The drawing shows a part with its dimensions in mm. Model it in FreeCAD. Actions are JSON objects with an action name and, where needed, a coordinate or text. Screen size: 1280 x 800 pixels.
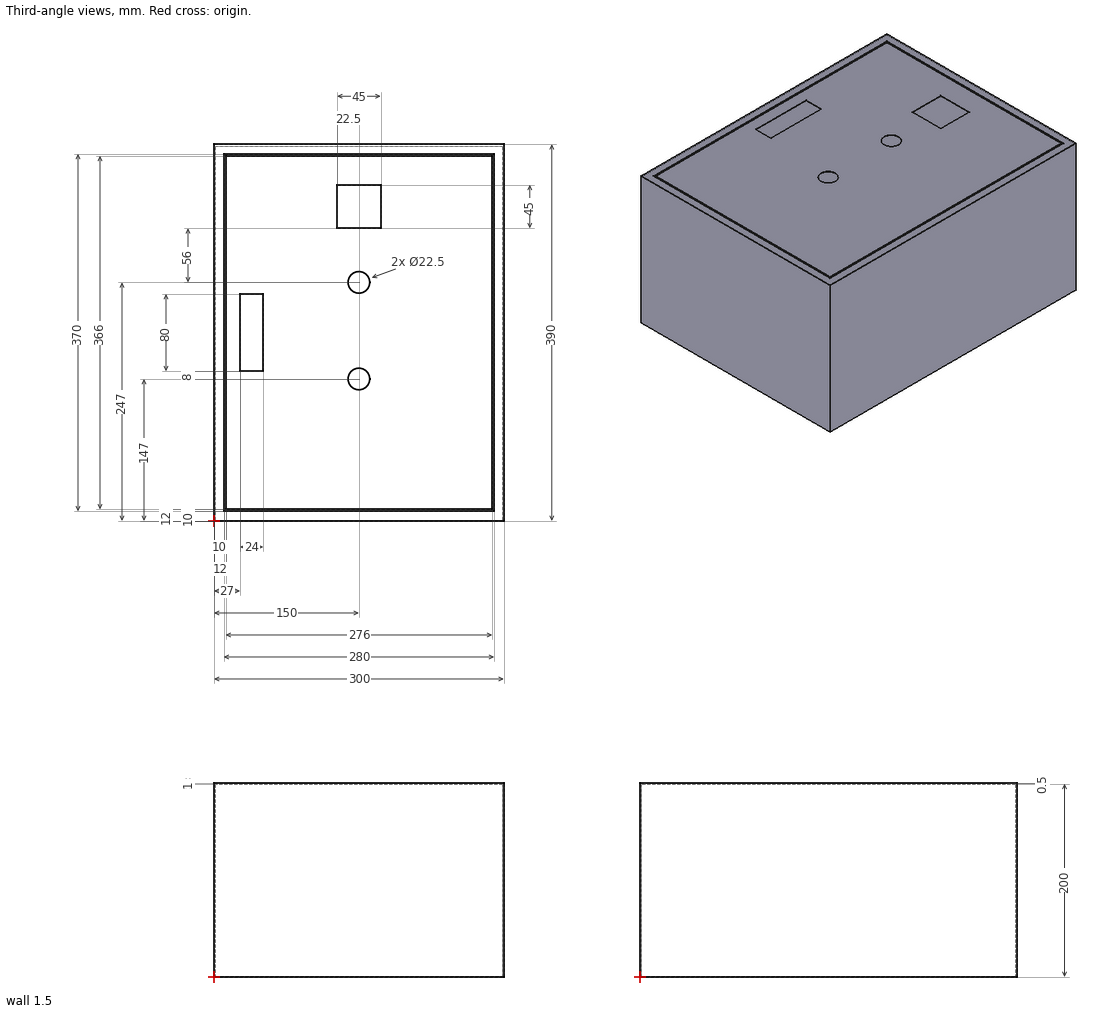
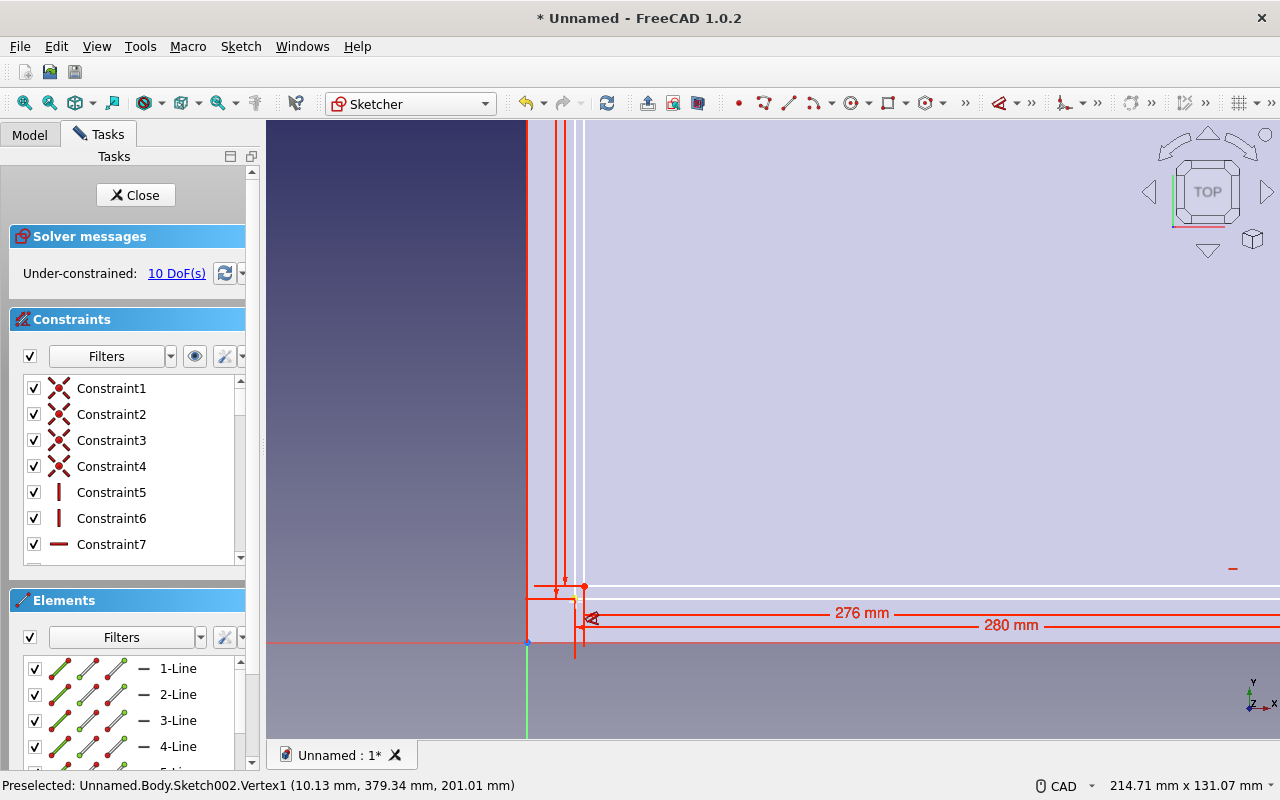
{"action": "left_click", "coordinate": [575, 599]}
{"action": "left_click", "coordinate": [493, 621]}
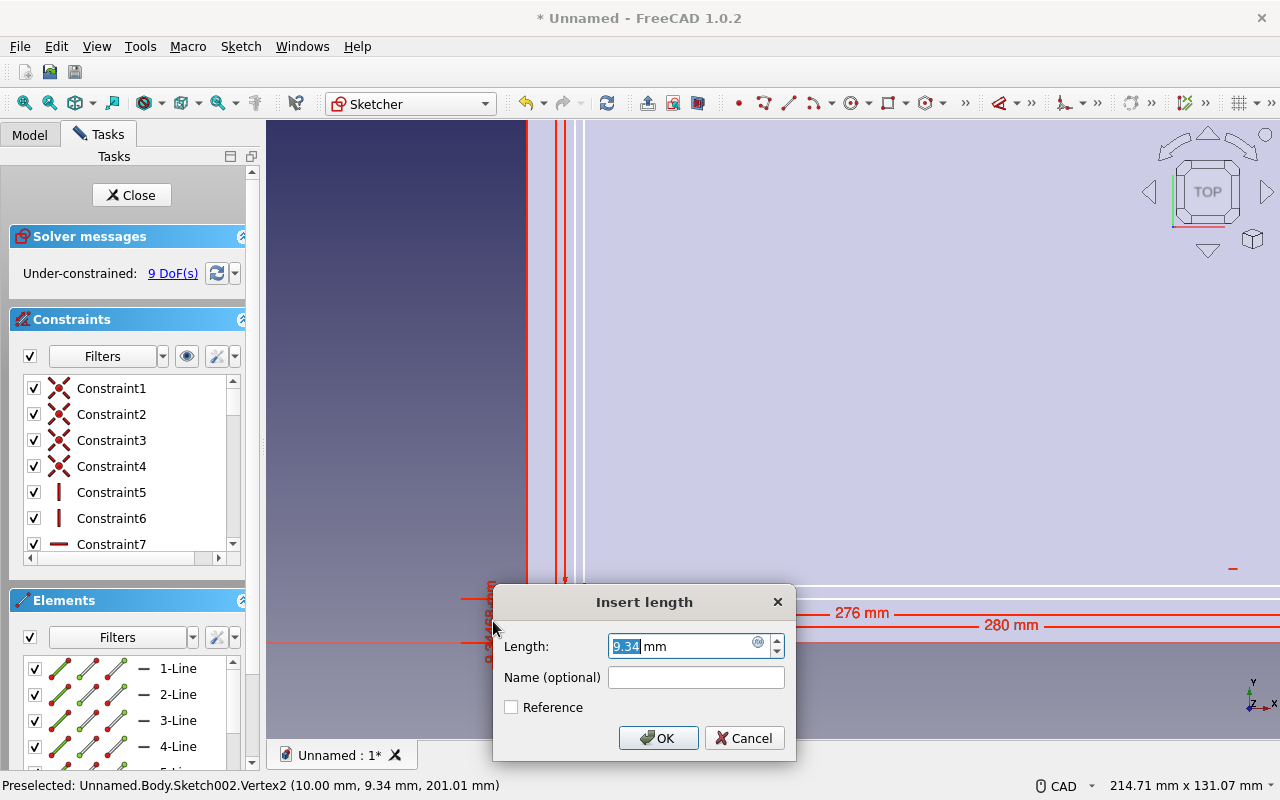
{"action": "type", "text": "10"}
{"action": "key", "text": "Return"}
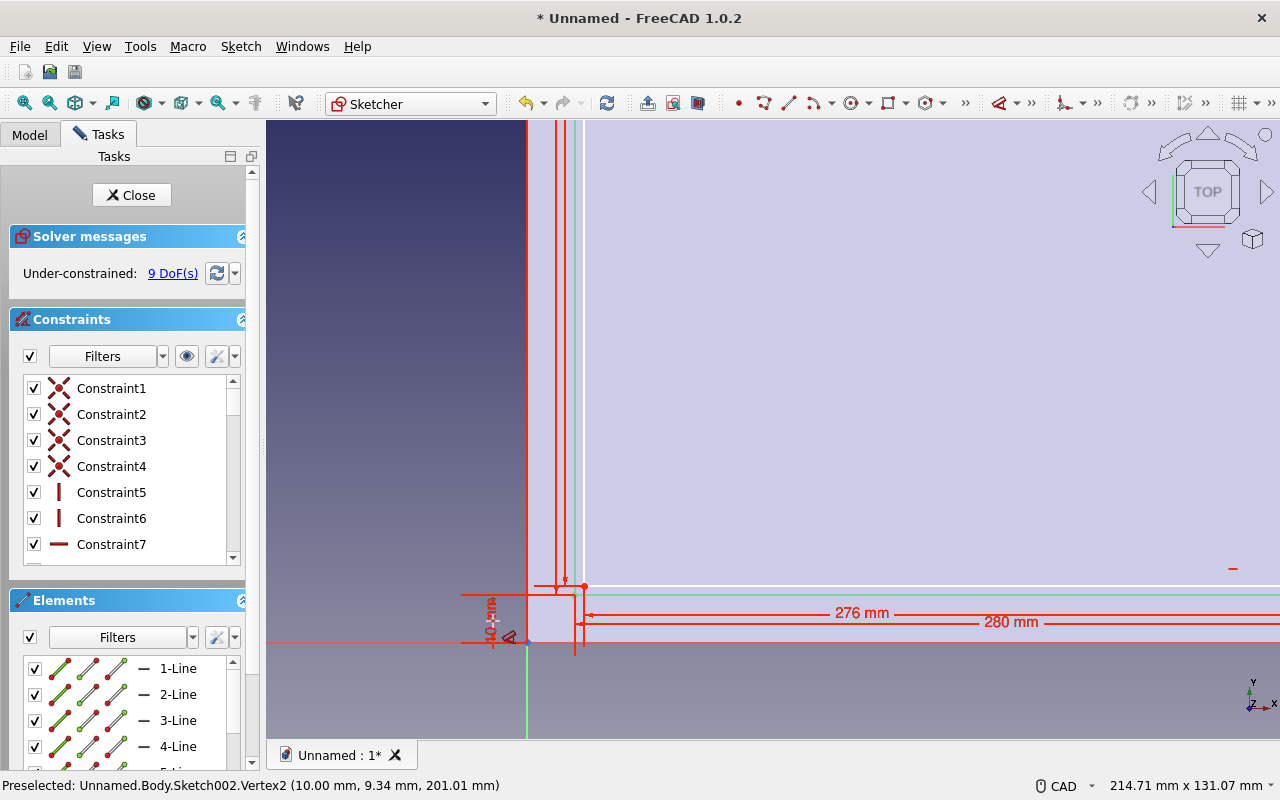
{"action": "scroll", "coordinate": [576, 603], "scroll_direction": "down", "scroll_amount": 8}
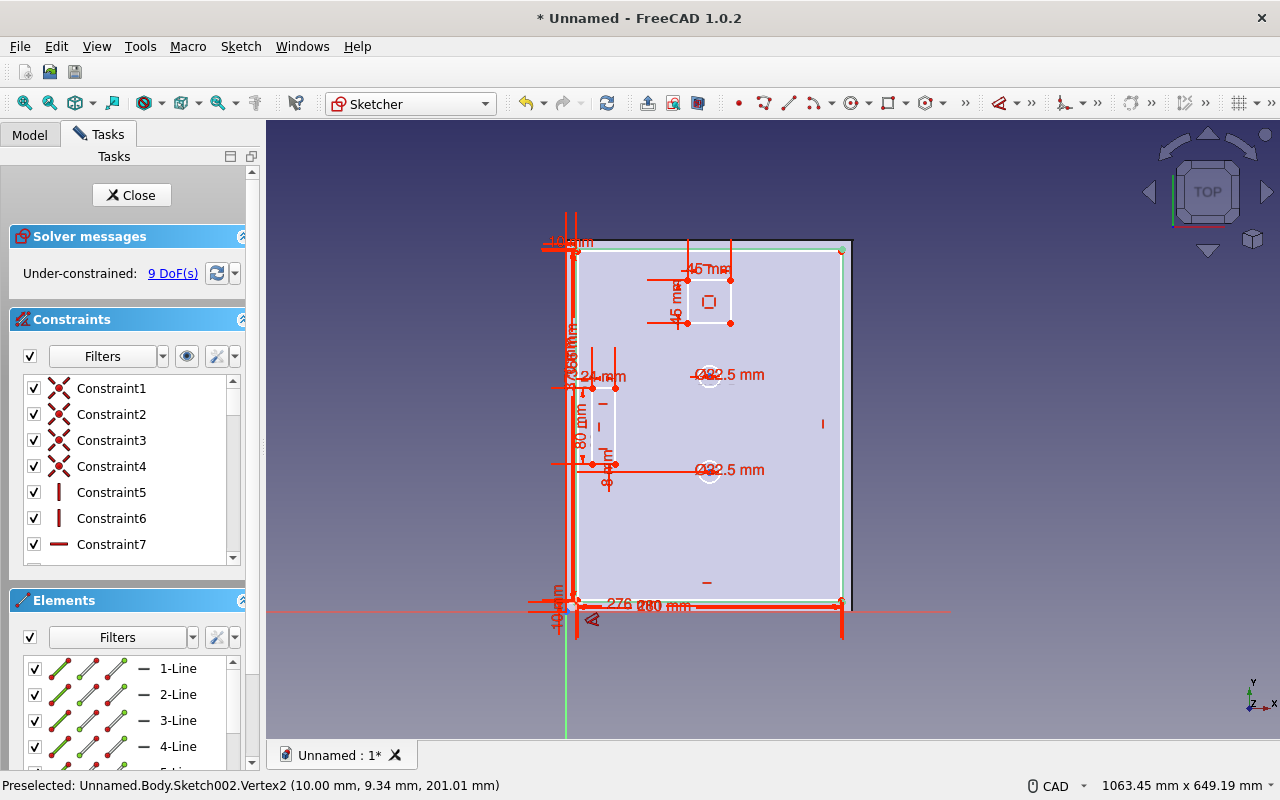
{"action": "scroll", "coordinate": [592, 388], "scroll_direction": "up", "scroll_amount": 3}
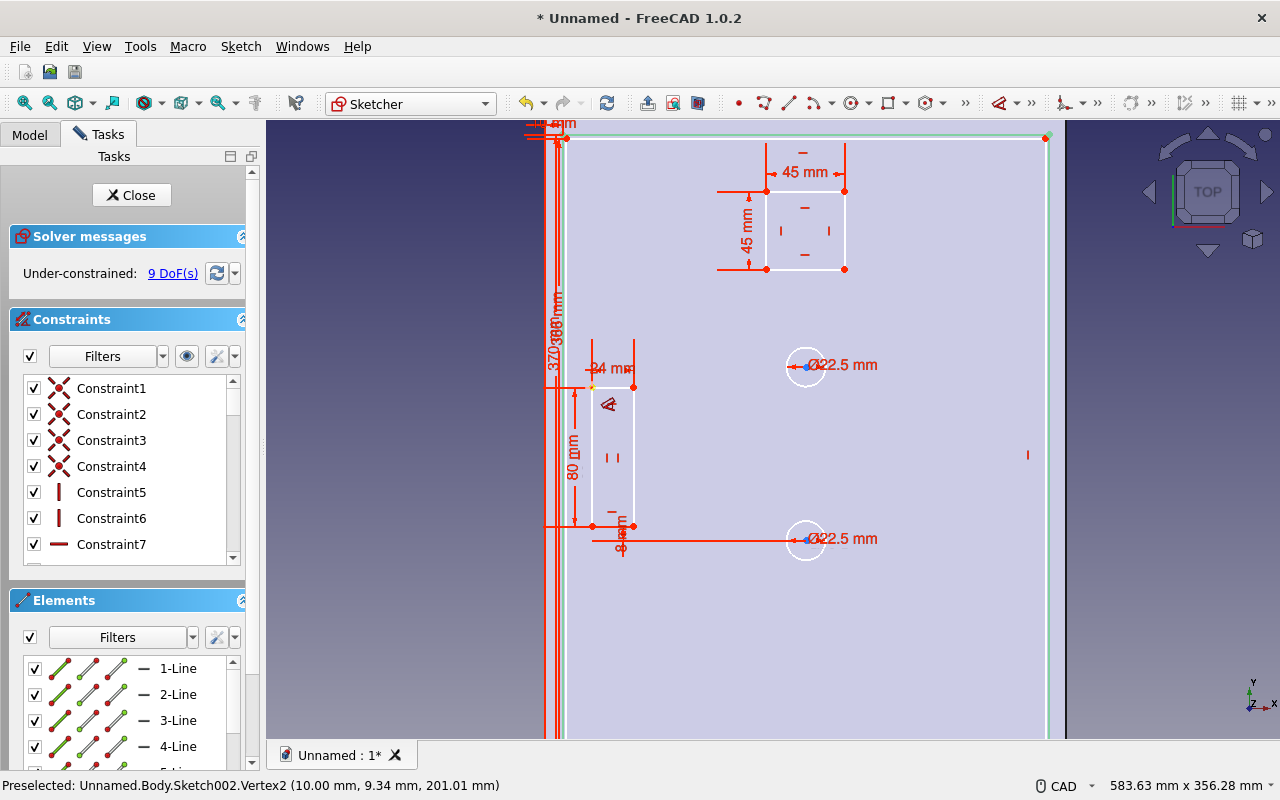
{"action": "left_click", "coordinate": [592, 388]}
{"action": "left_click", "coordinate": [579, 282]}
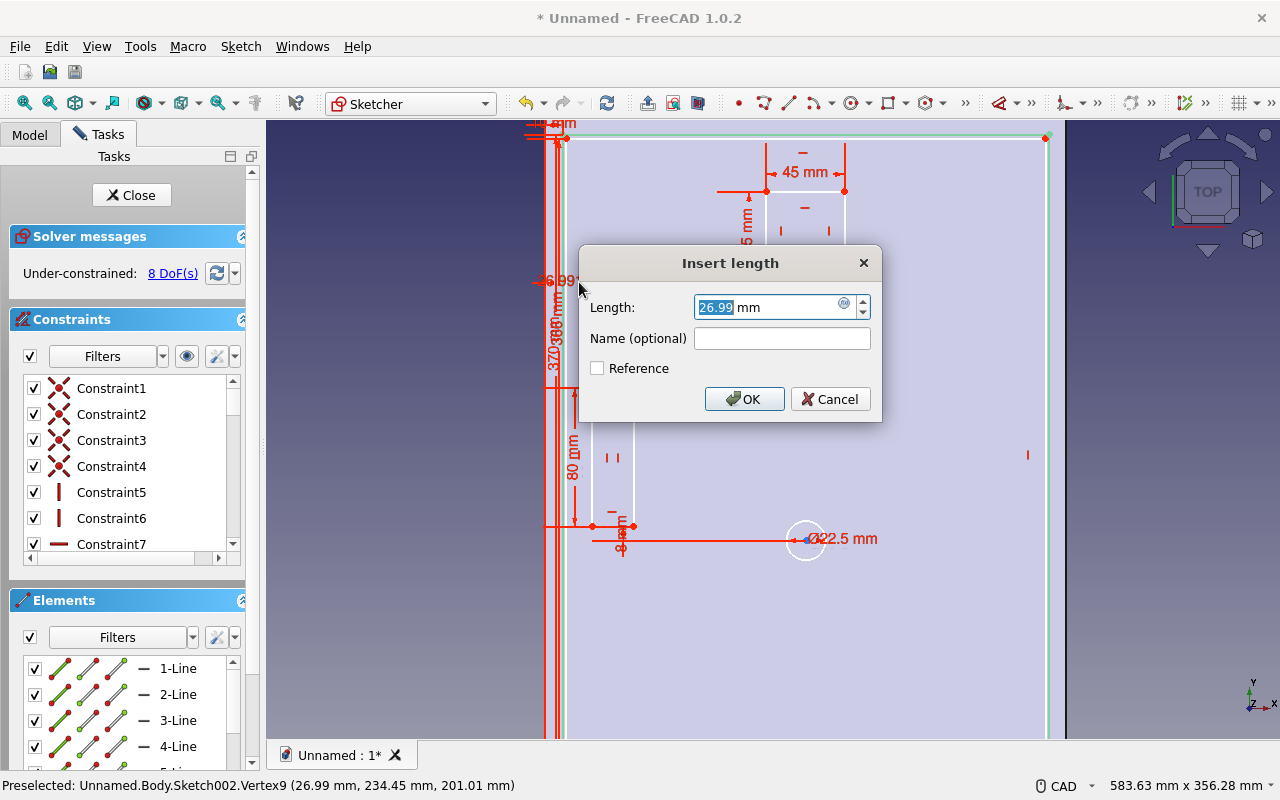
{"action": "type", "text": "27"}
{"action": "key", "text": "Return"}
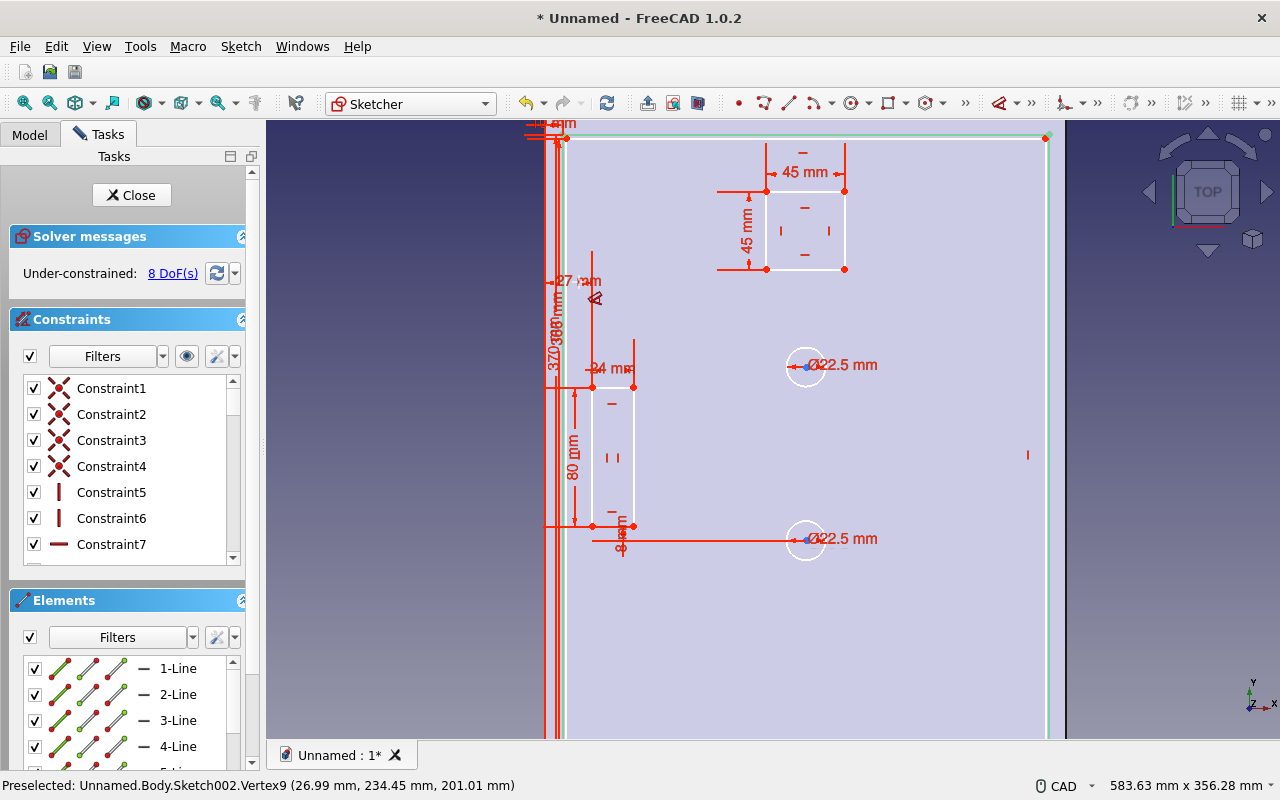
{"action": "scroll", "coordinate": [592, 386], "scroll_direction": "down", "scroll_amount": 3}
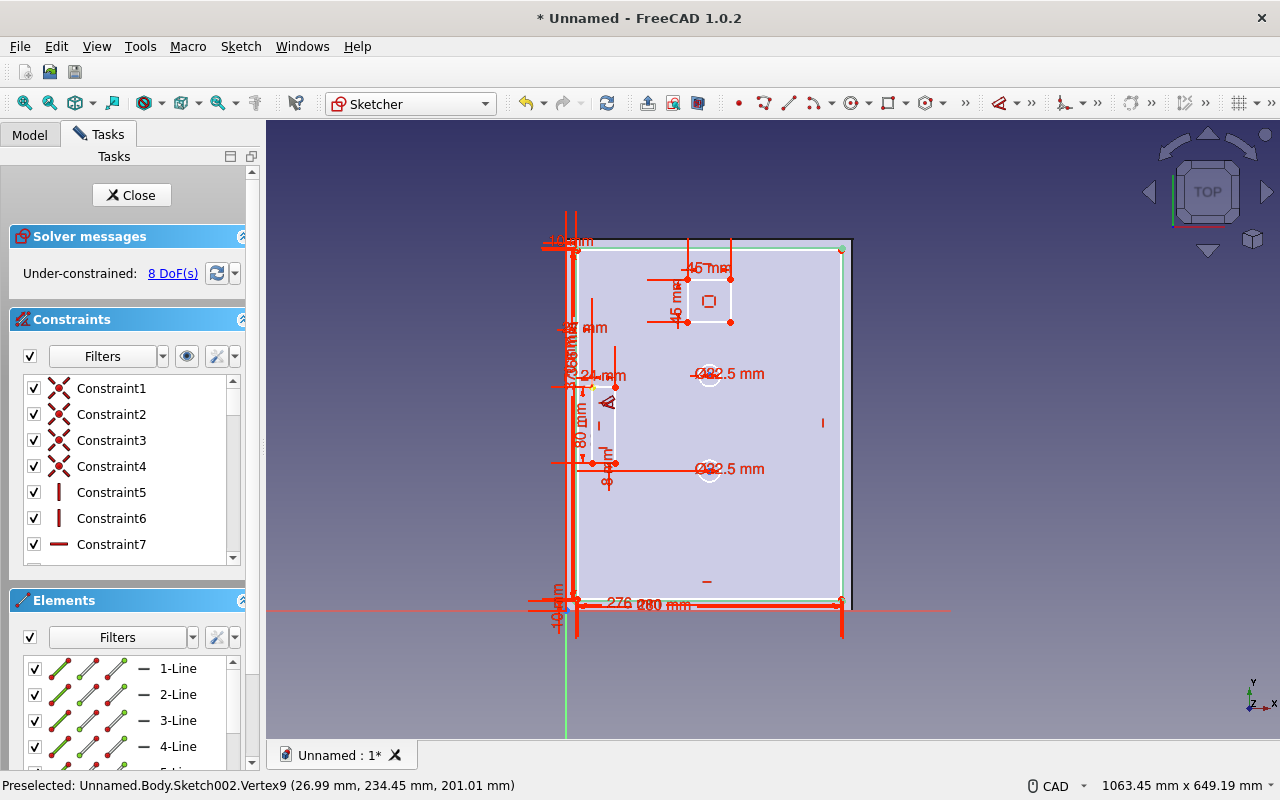
{"action": "scroll", "coordinate": [578, 250], "scroll_direction": "up", "scroll_amount": 8}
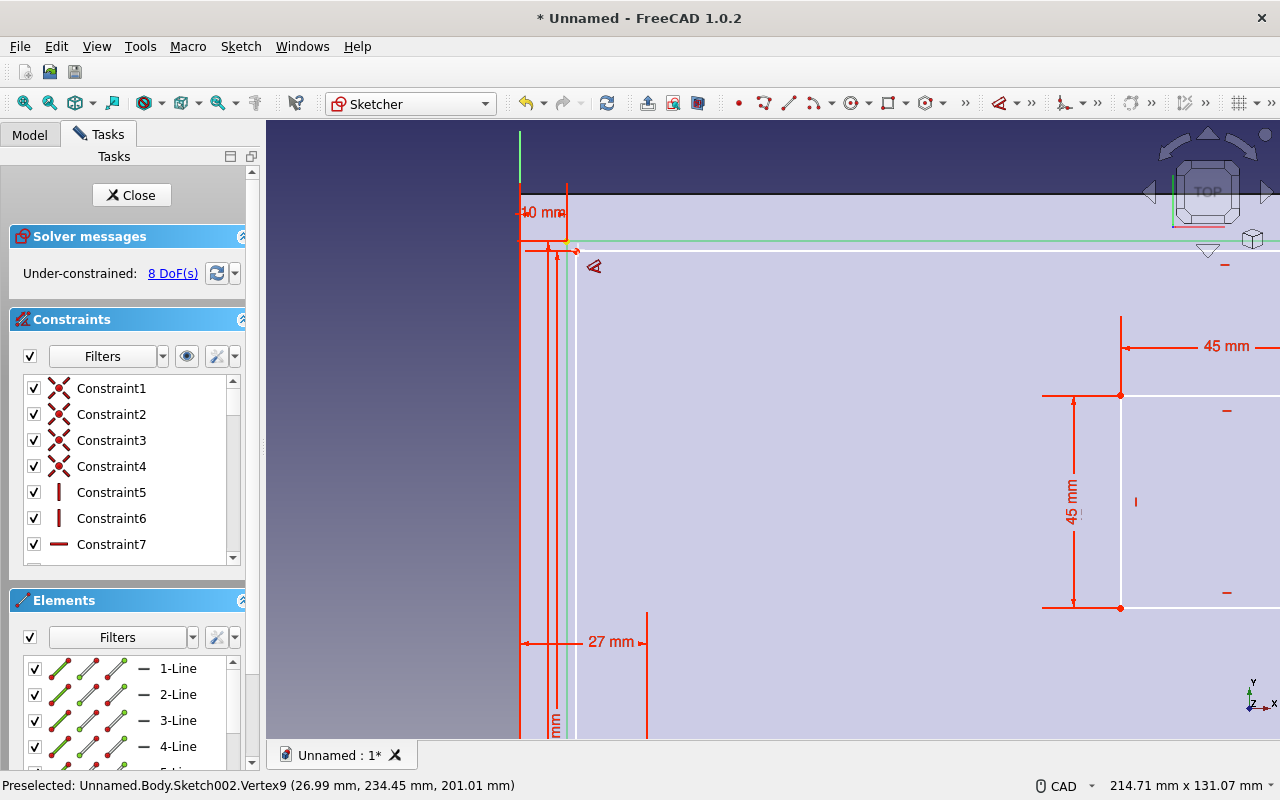
{"action": "left_click", "coordinate": [576, 251]}
{"action": "left_click", "coordinate": [548, 193]}